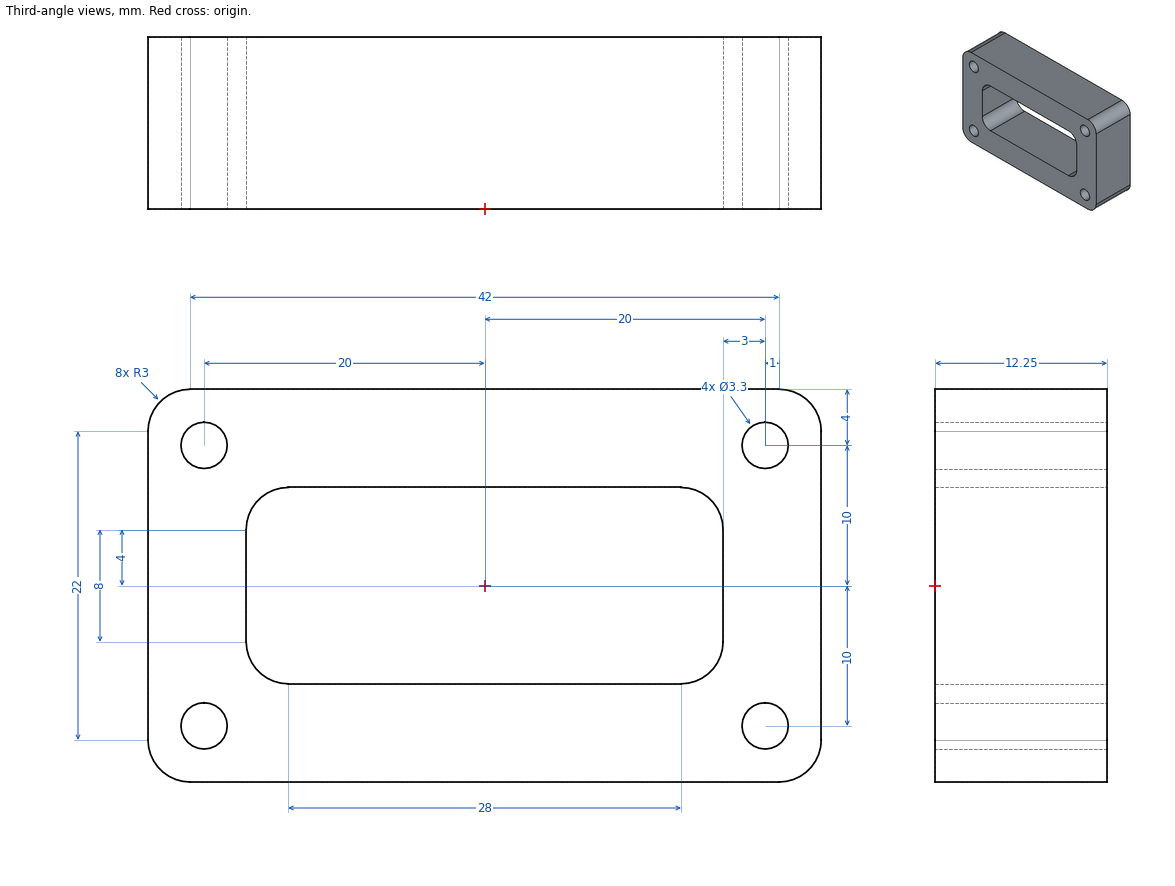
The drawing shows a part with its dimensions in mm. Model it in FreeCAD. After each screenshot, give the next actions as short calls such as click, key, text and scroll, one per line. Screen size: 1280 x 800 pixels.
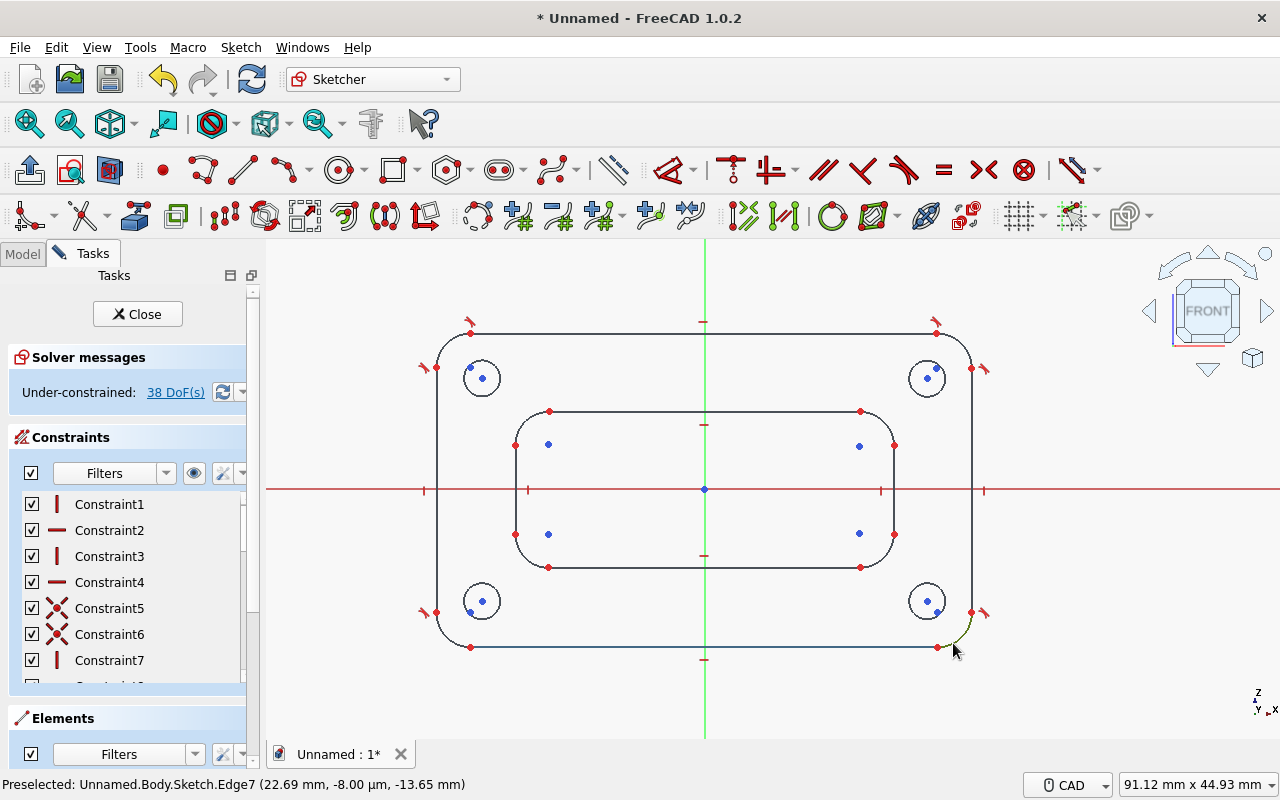
click(904, 170)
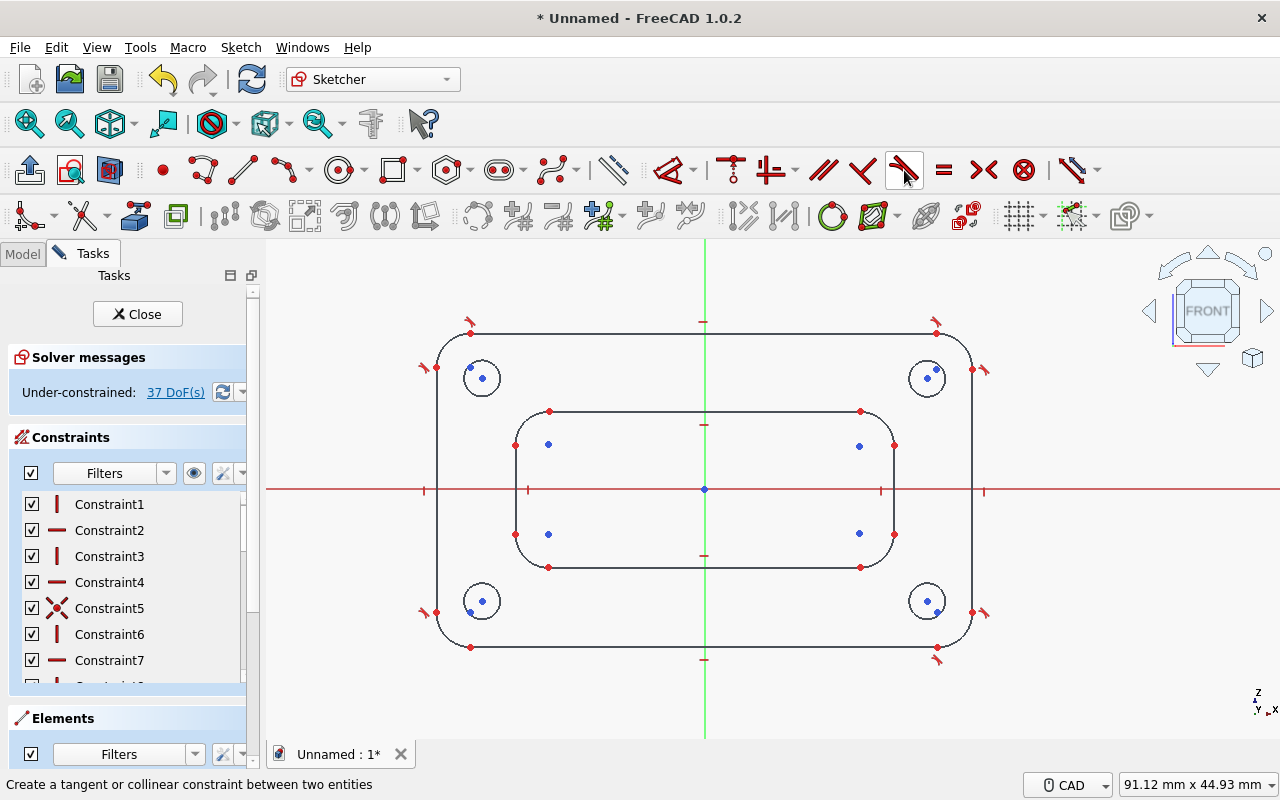
click(798, 647)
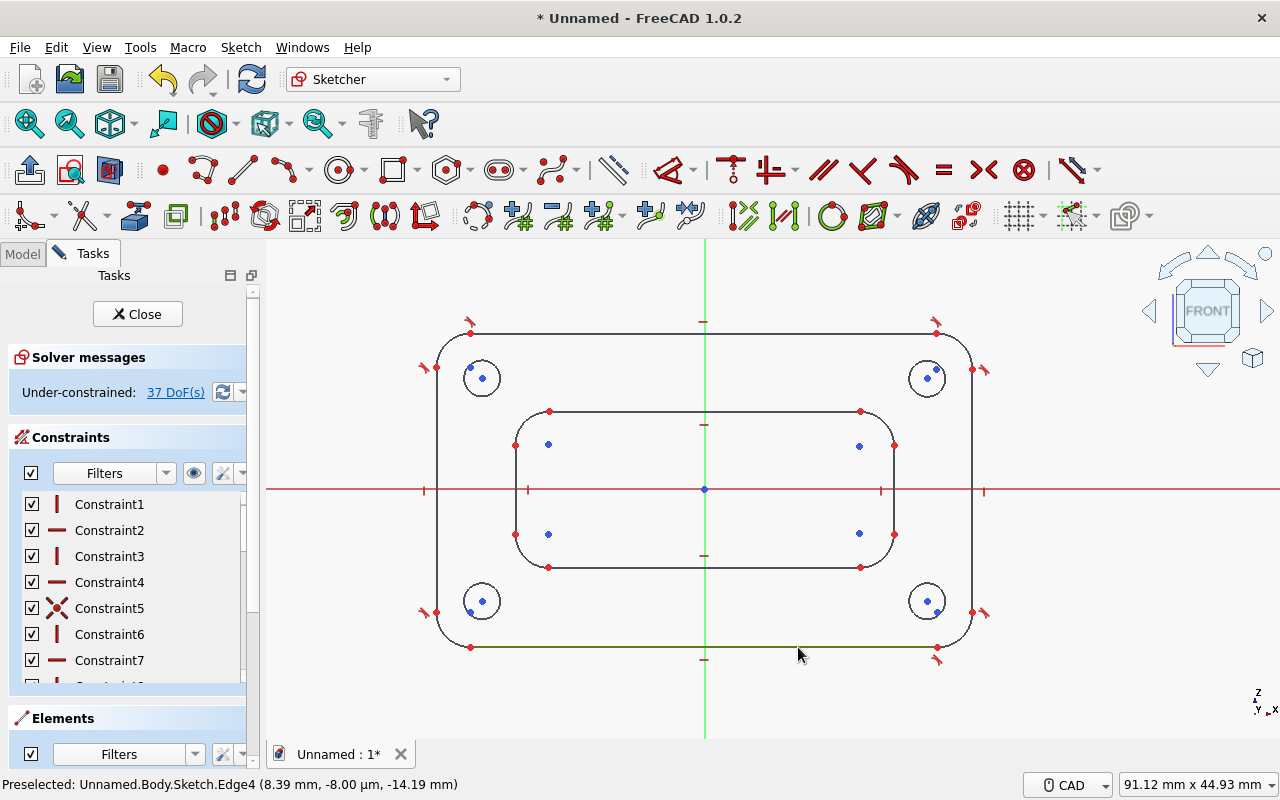
click(440, 628)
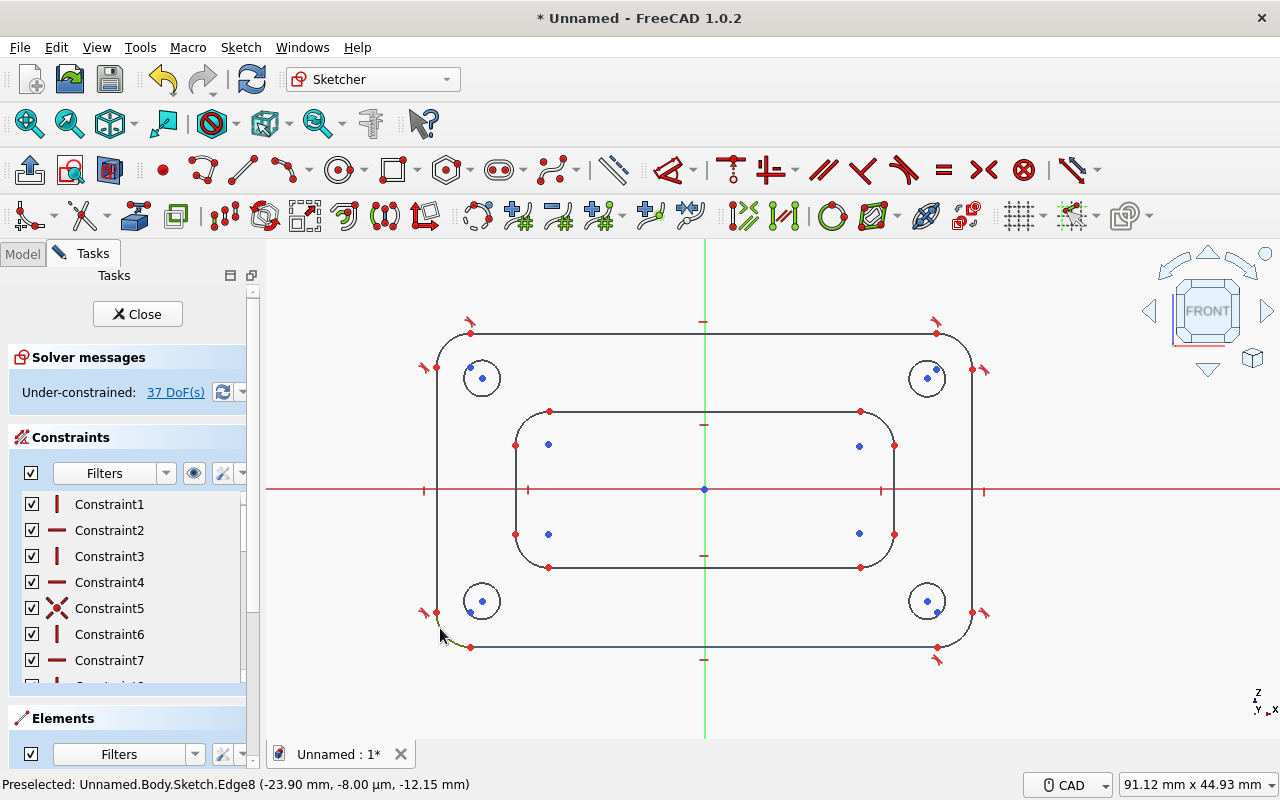
click(904, 170)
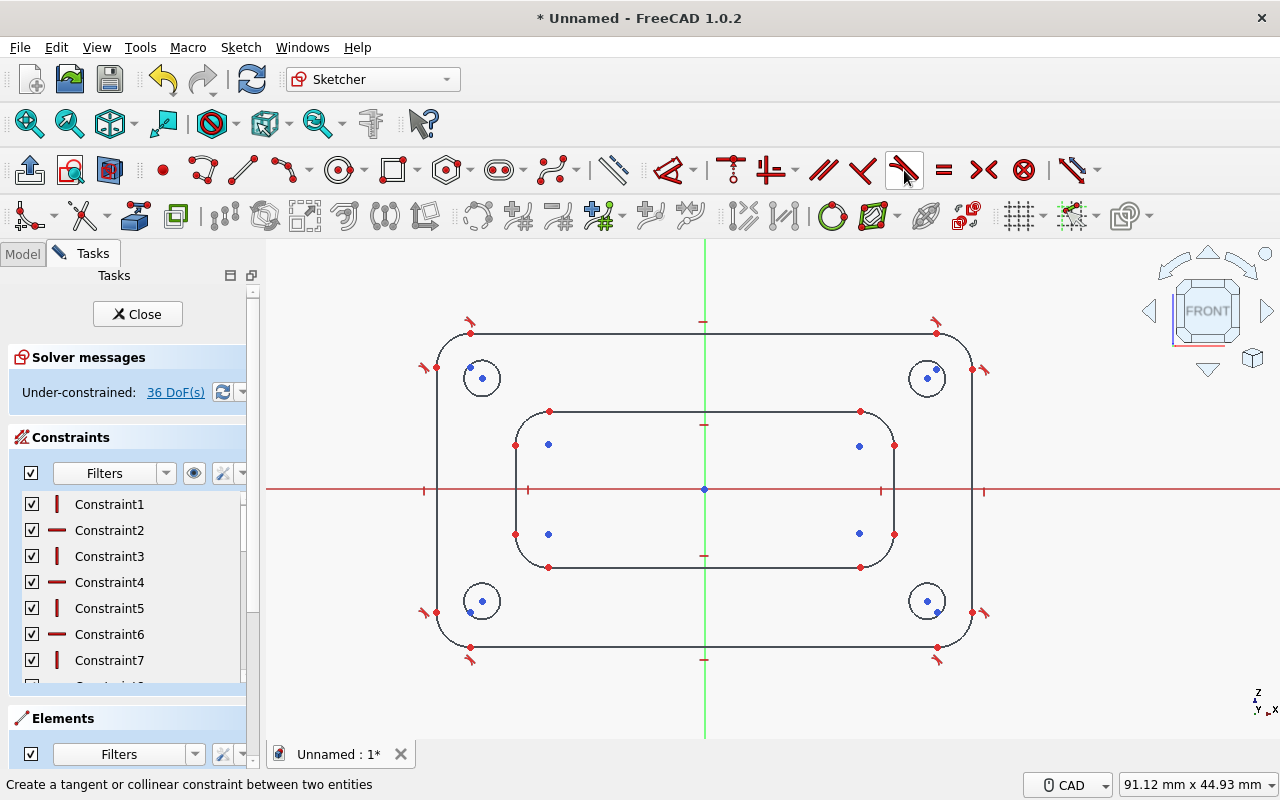
click(516, 472)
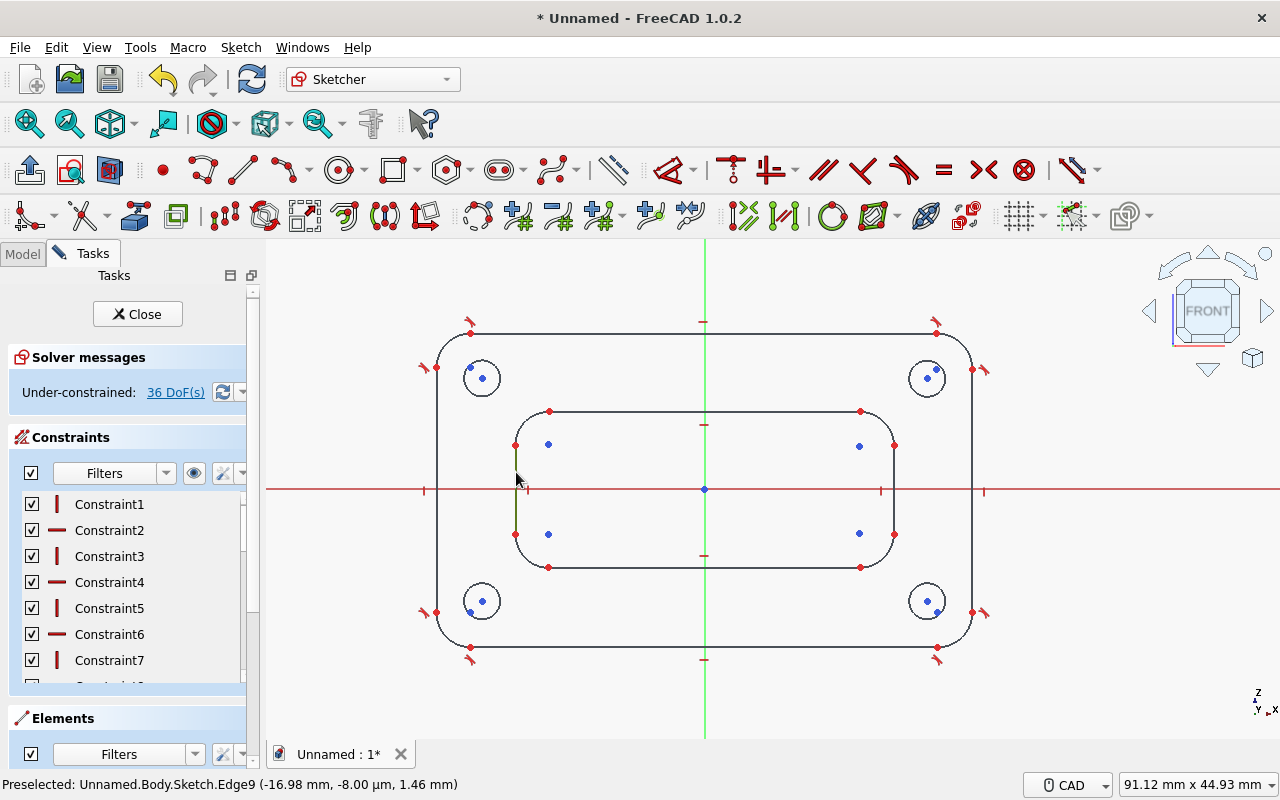
click(519, 549)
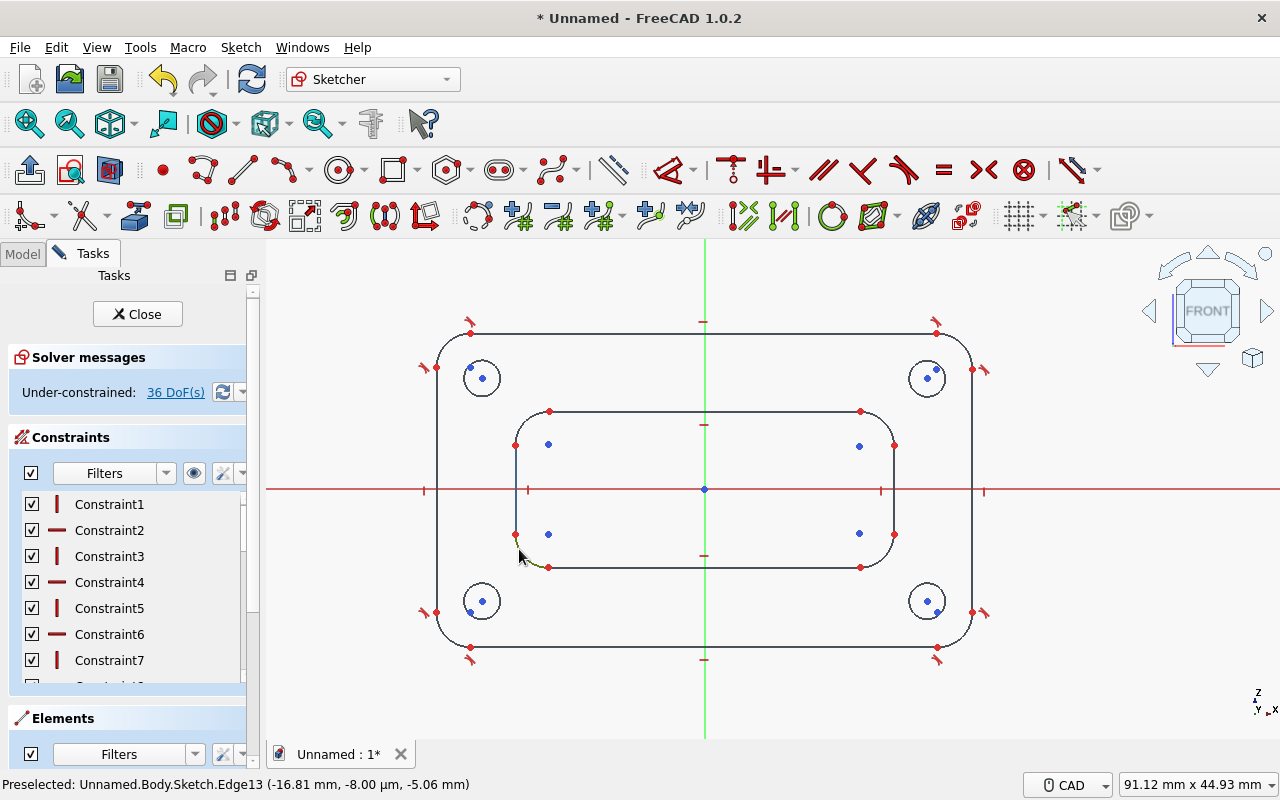
click(904, 170)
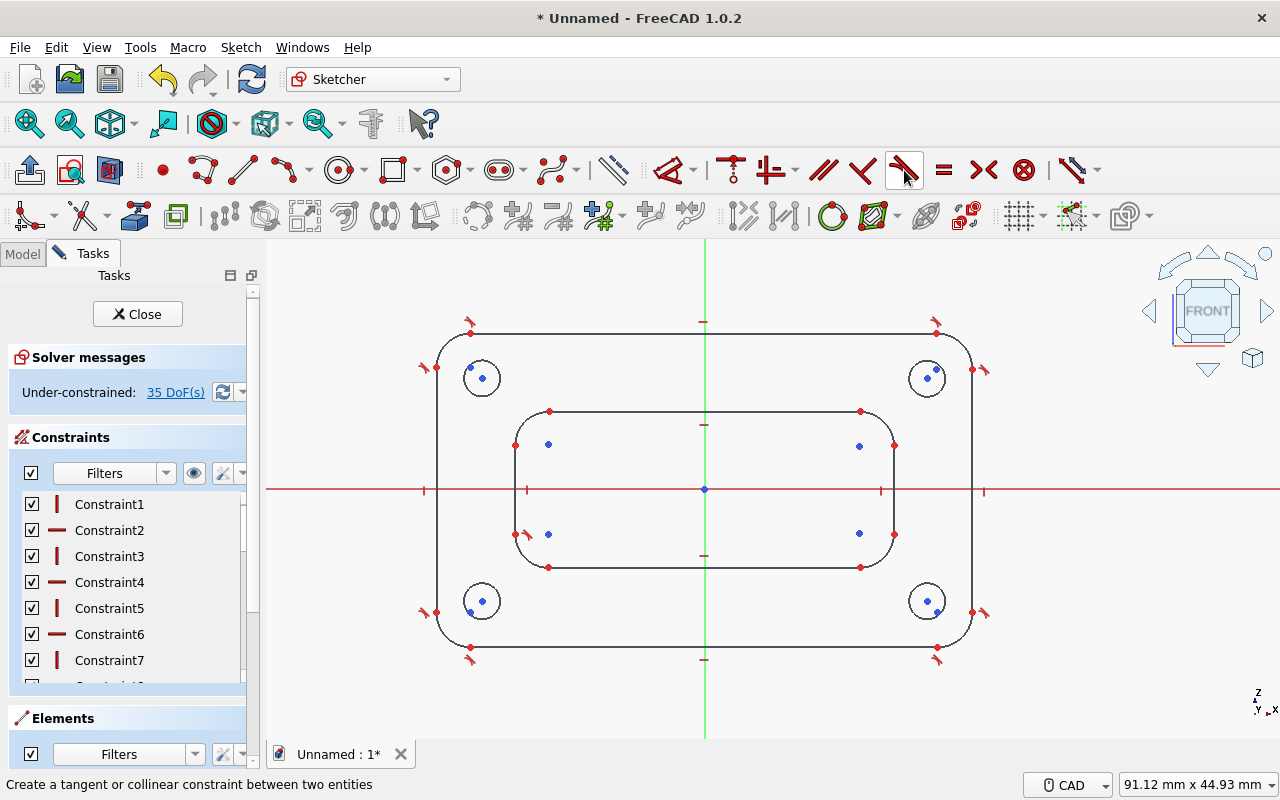
click(515, 472)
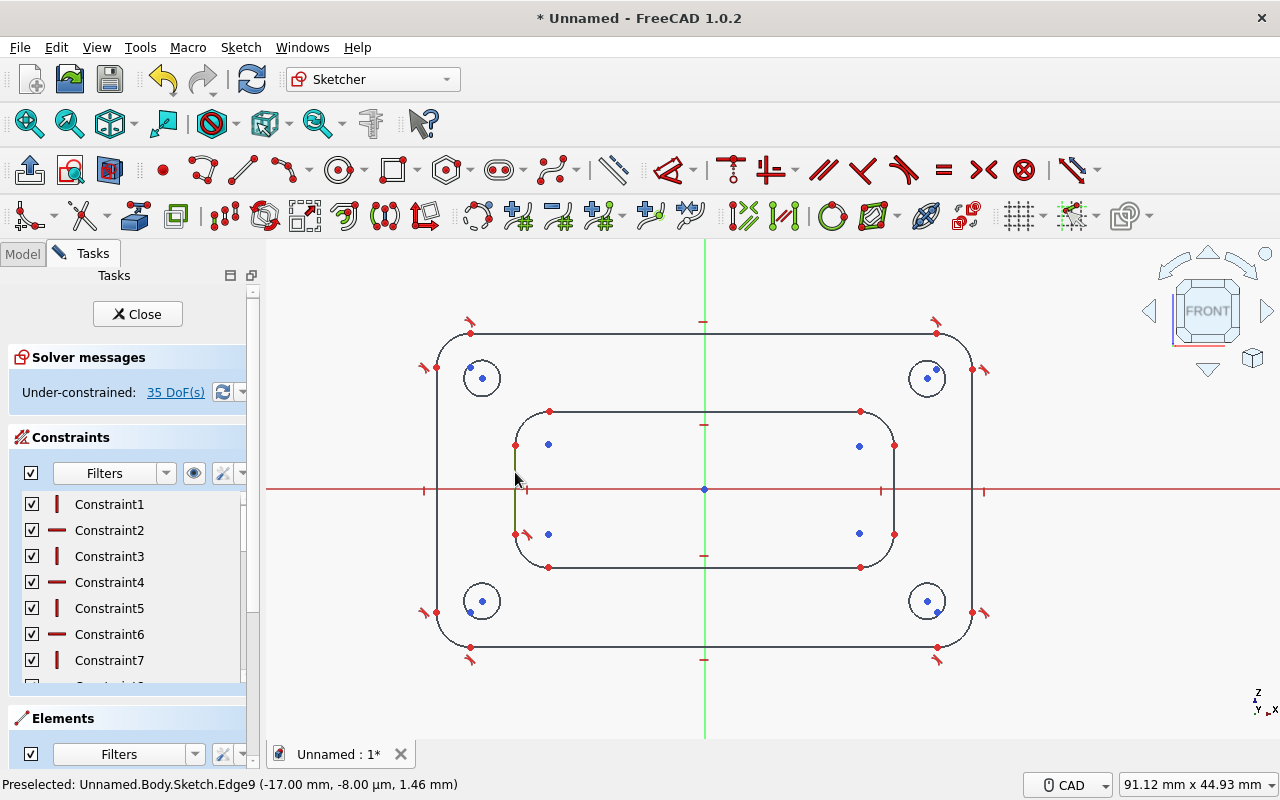
click(534, 415)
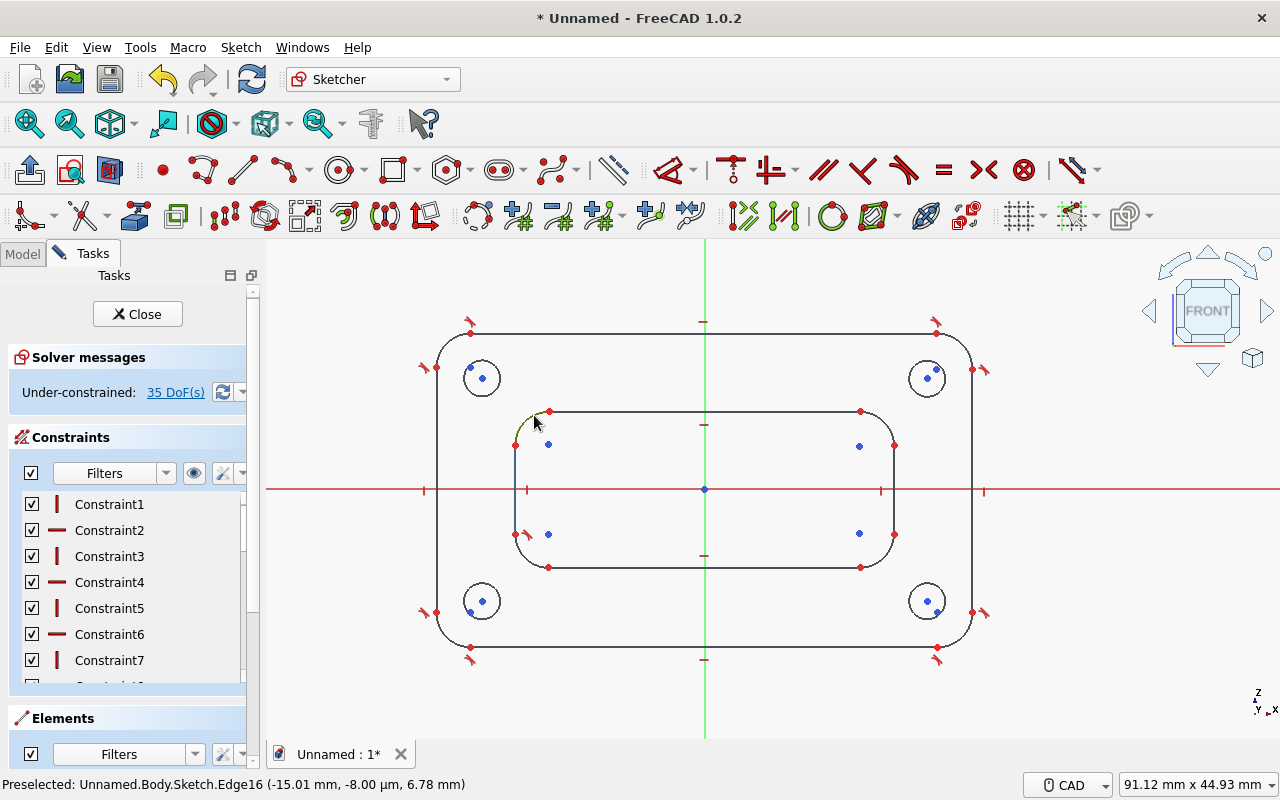
click(904, 170)